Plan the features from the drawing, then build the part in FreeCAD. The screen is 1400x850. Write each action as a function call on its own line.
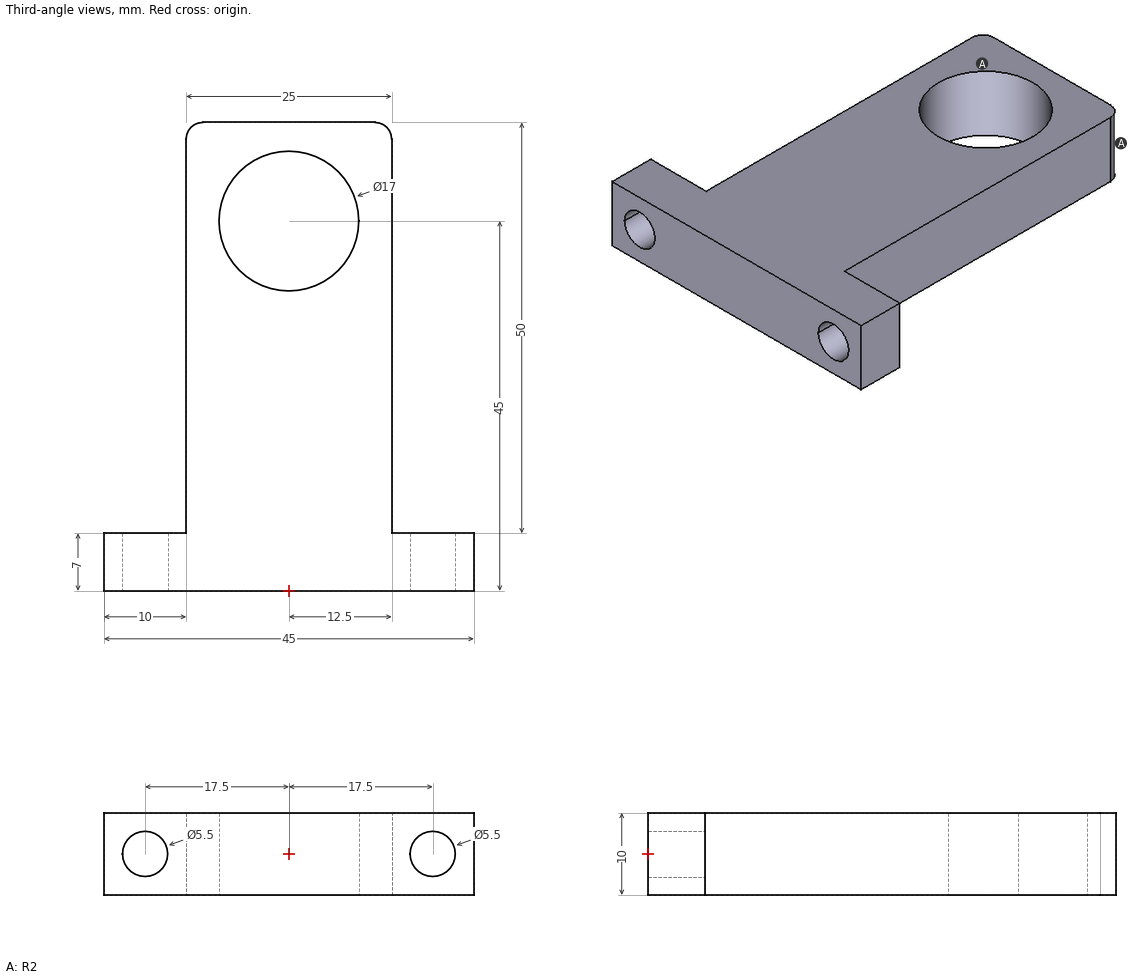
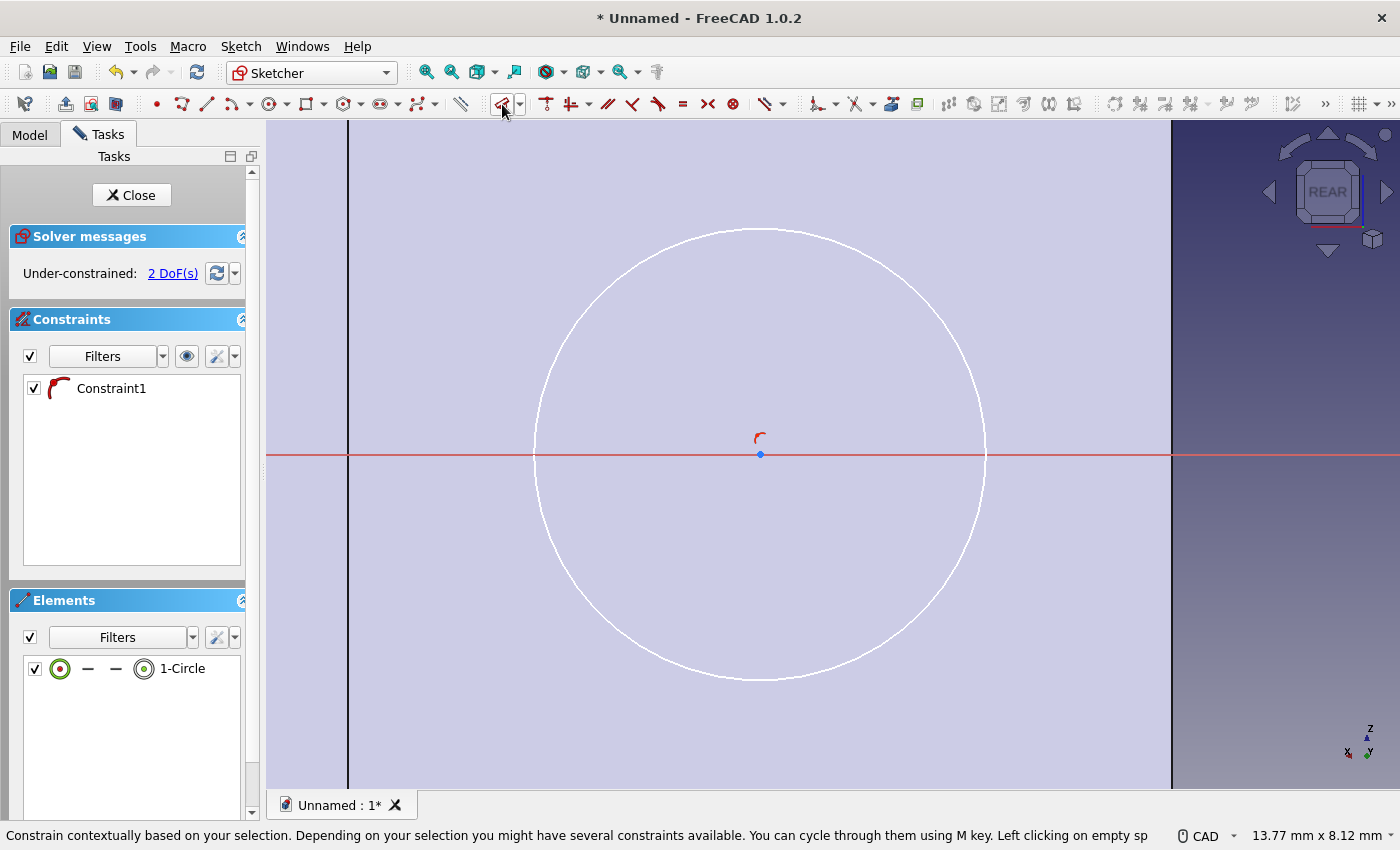
click(919, 294)
click(942, 271)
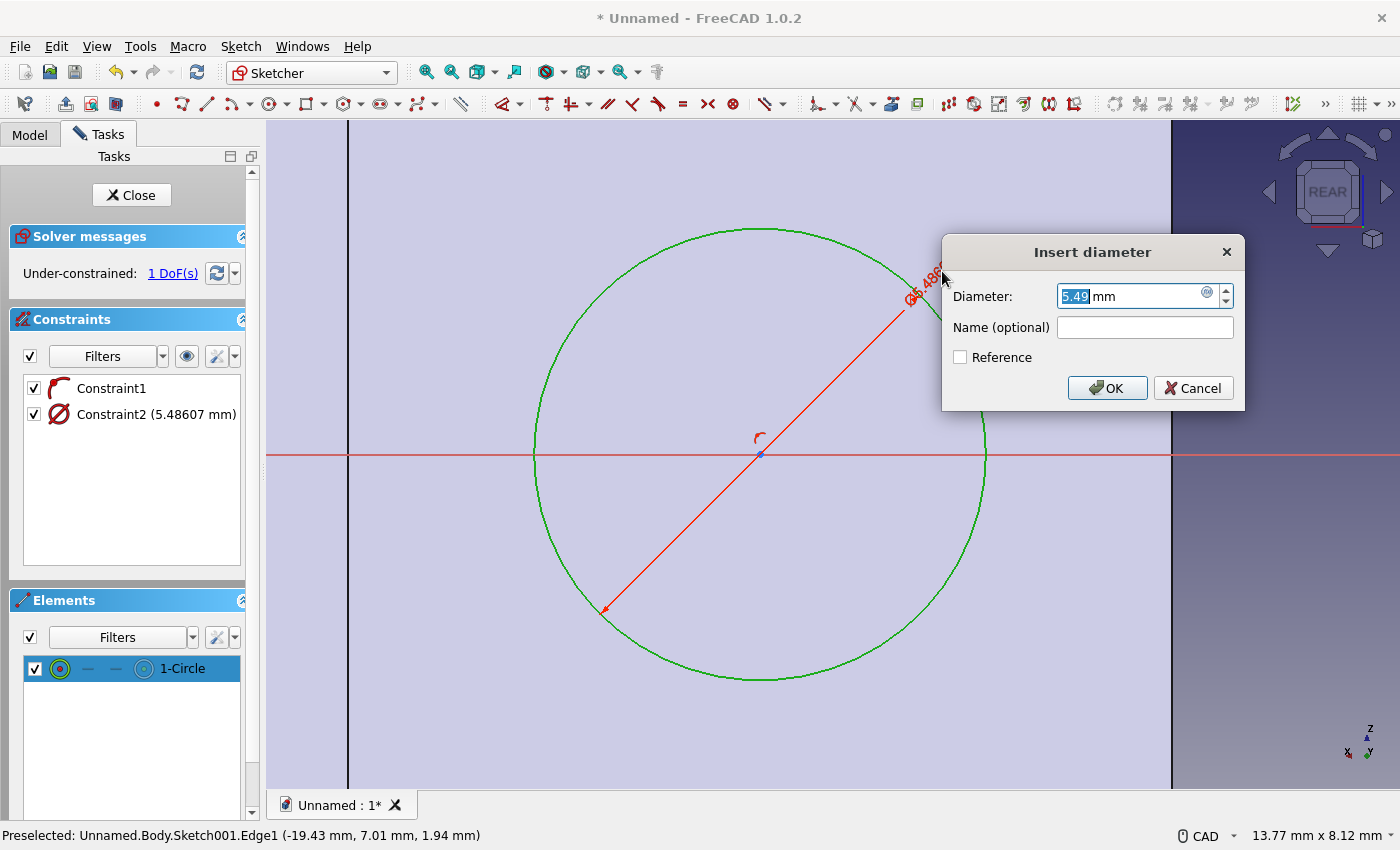
text(5.5)
key(Return)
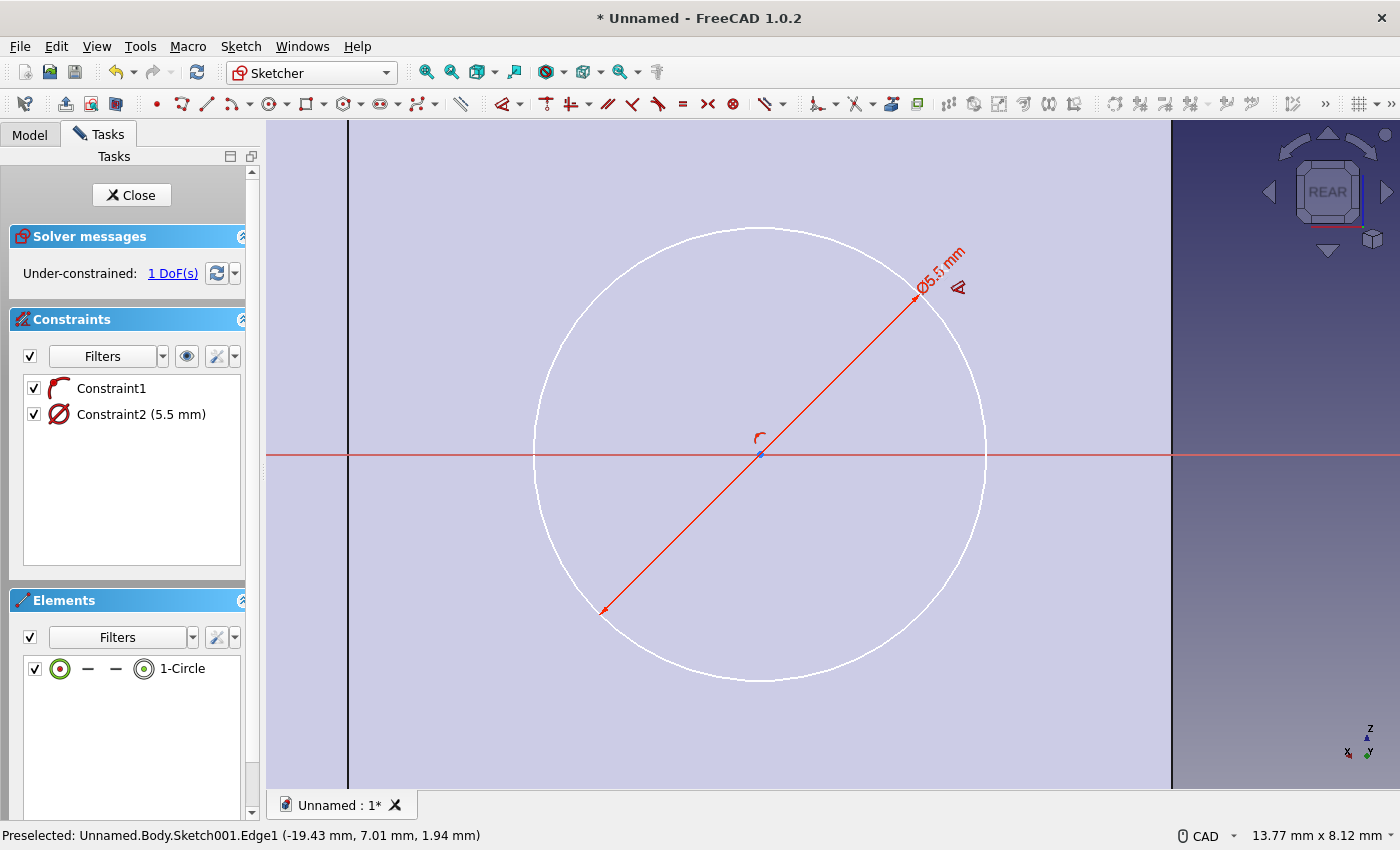
click(760, 454)
click(420, 488)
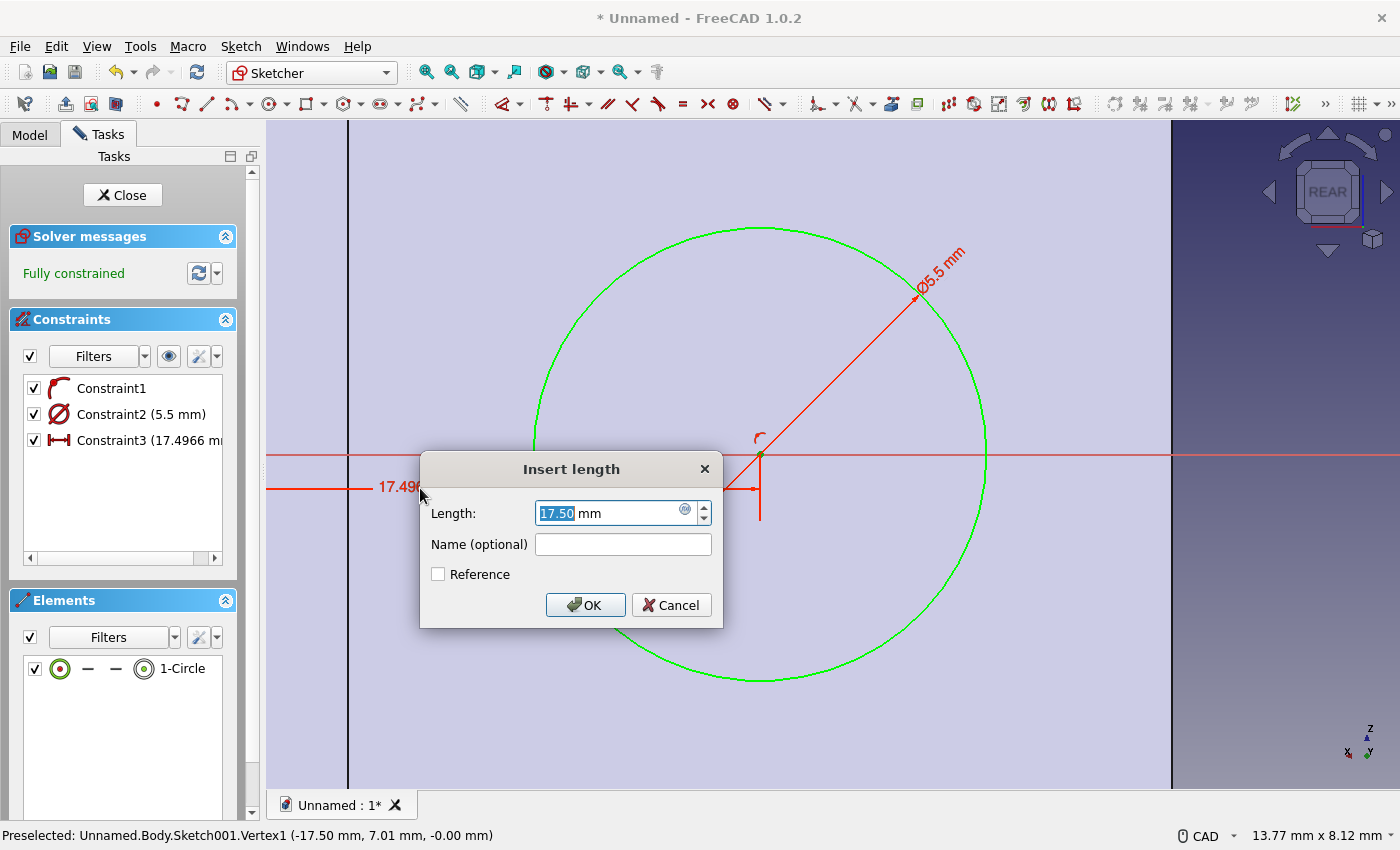
text(17.5)
key(Return)
key(Escape)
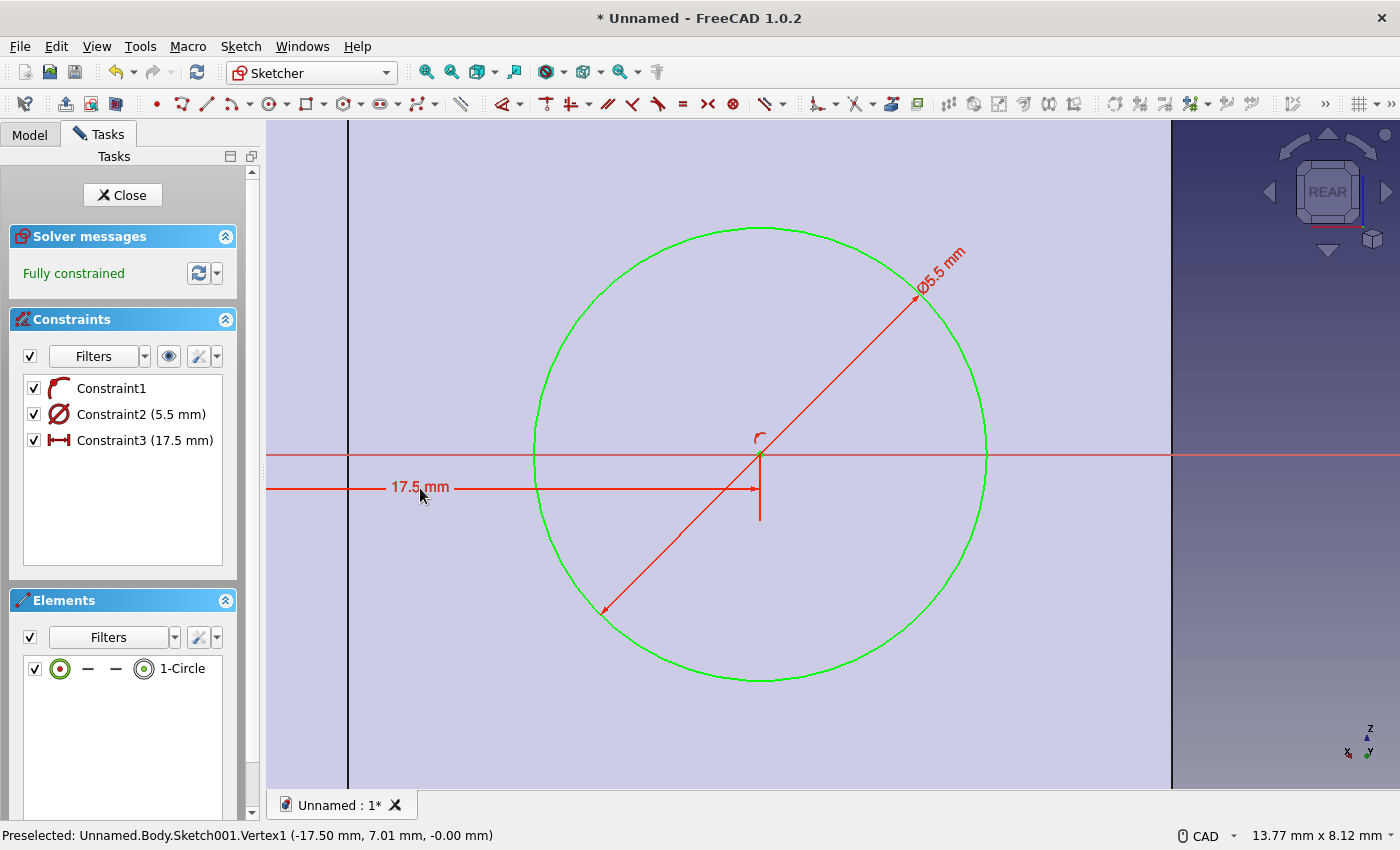
click(123, 195)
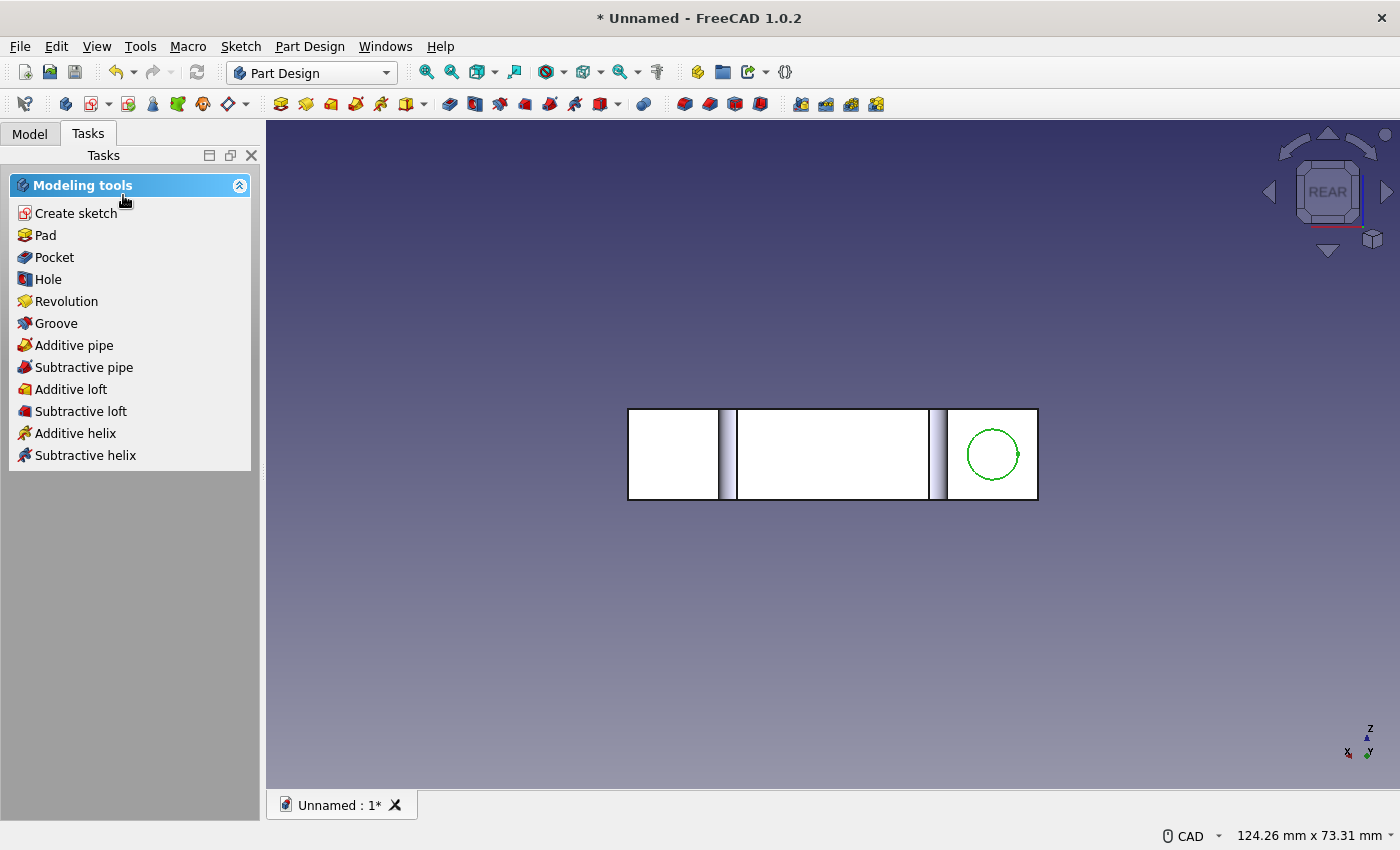
click(450, 104)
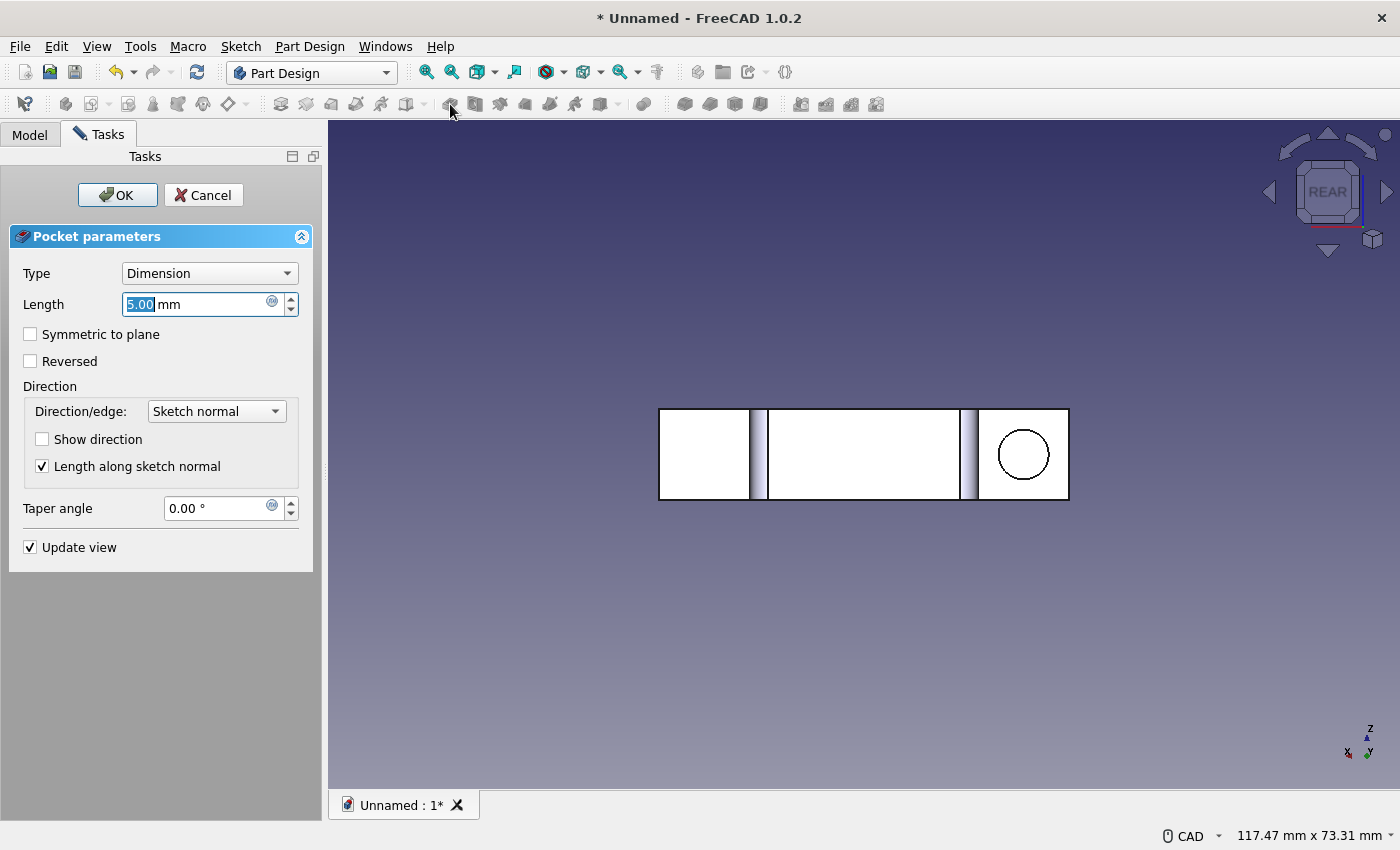
click(210, 274)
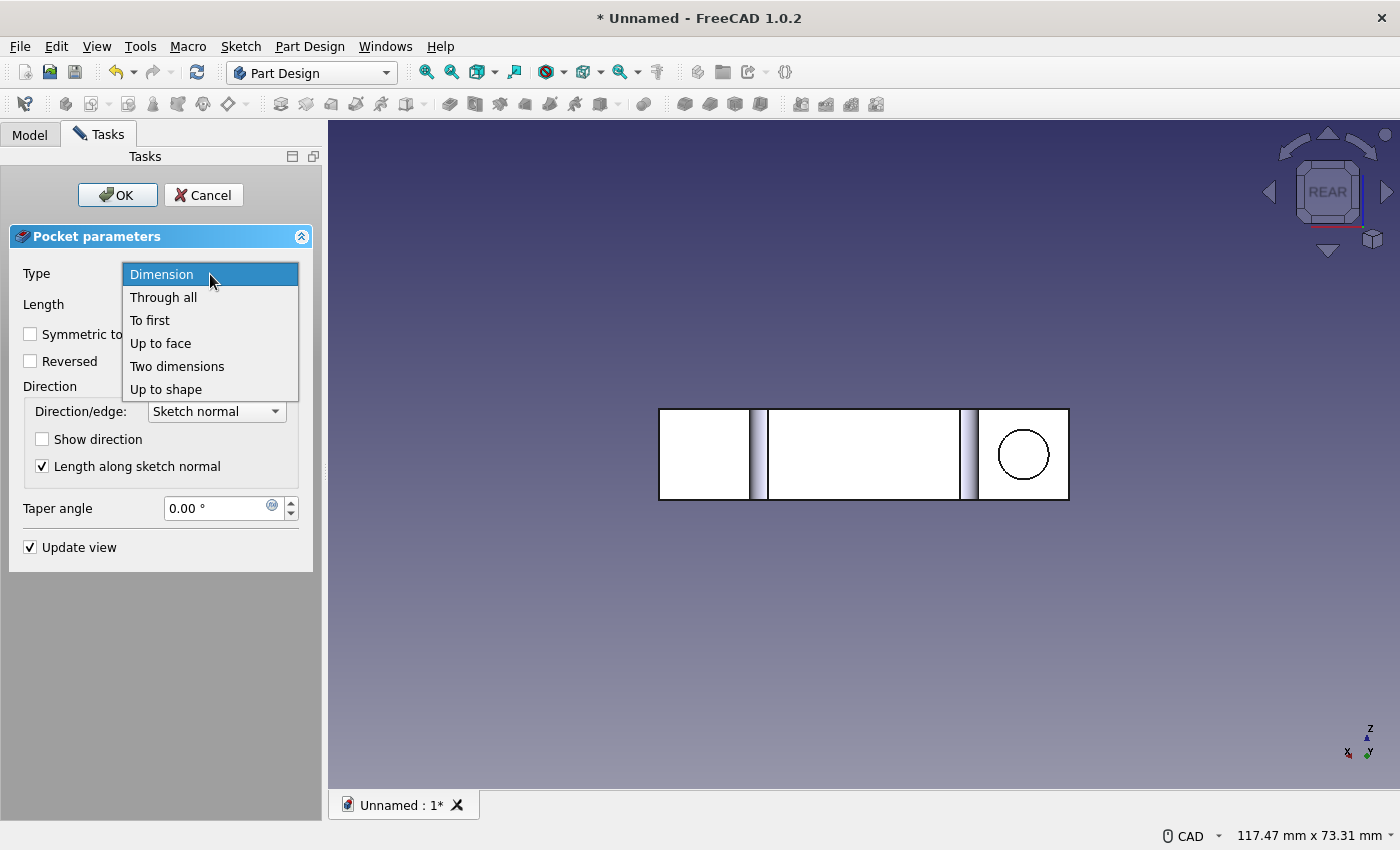
click(208, 320)